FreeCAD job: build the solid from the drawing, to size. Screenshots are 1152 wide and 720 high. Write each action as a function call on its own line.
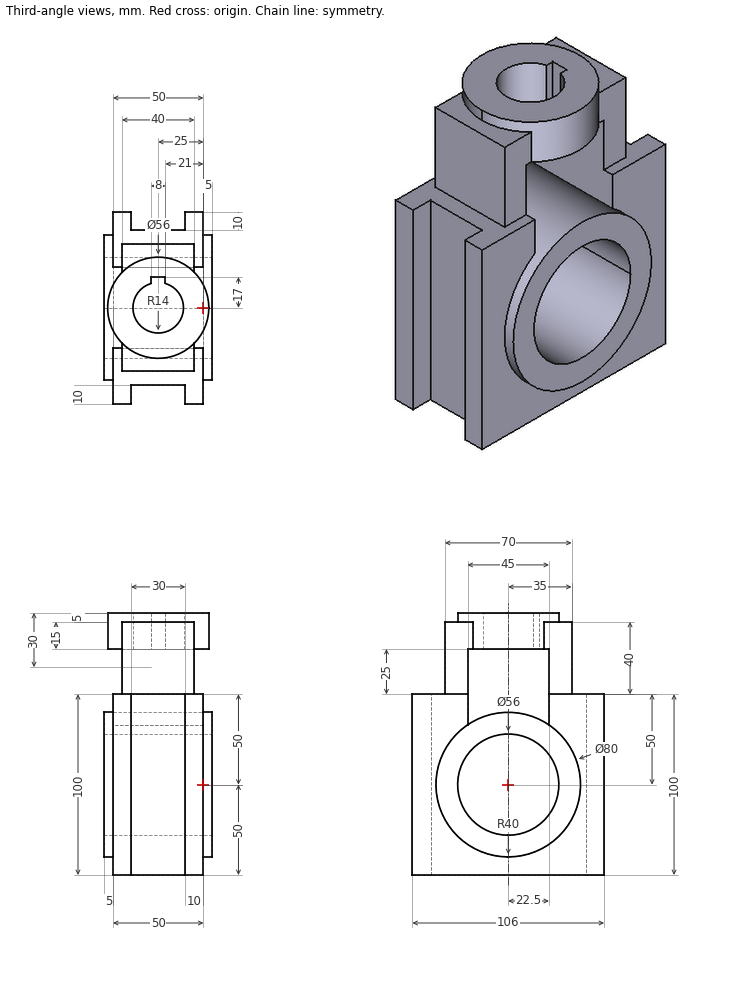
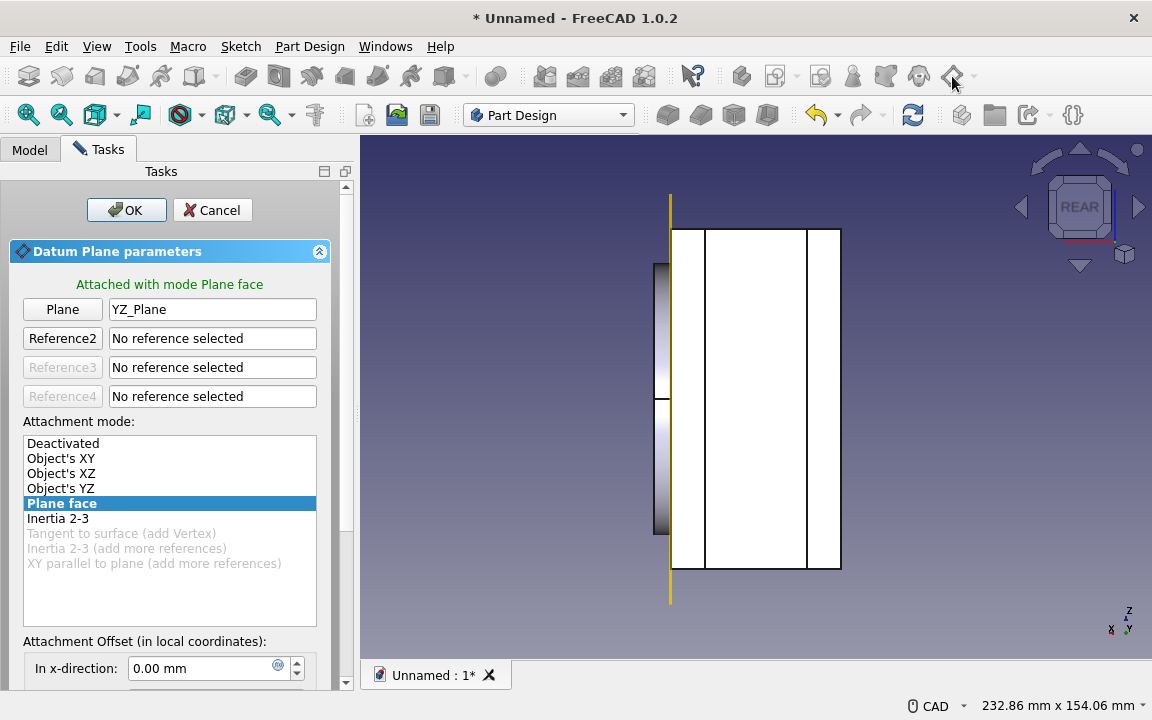
scroll(346, 436, down, 2)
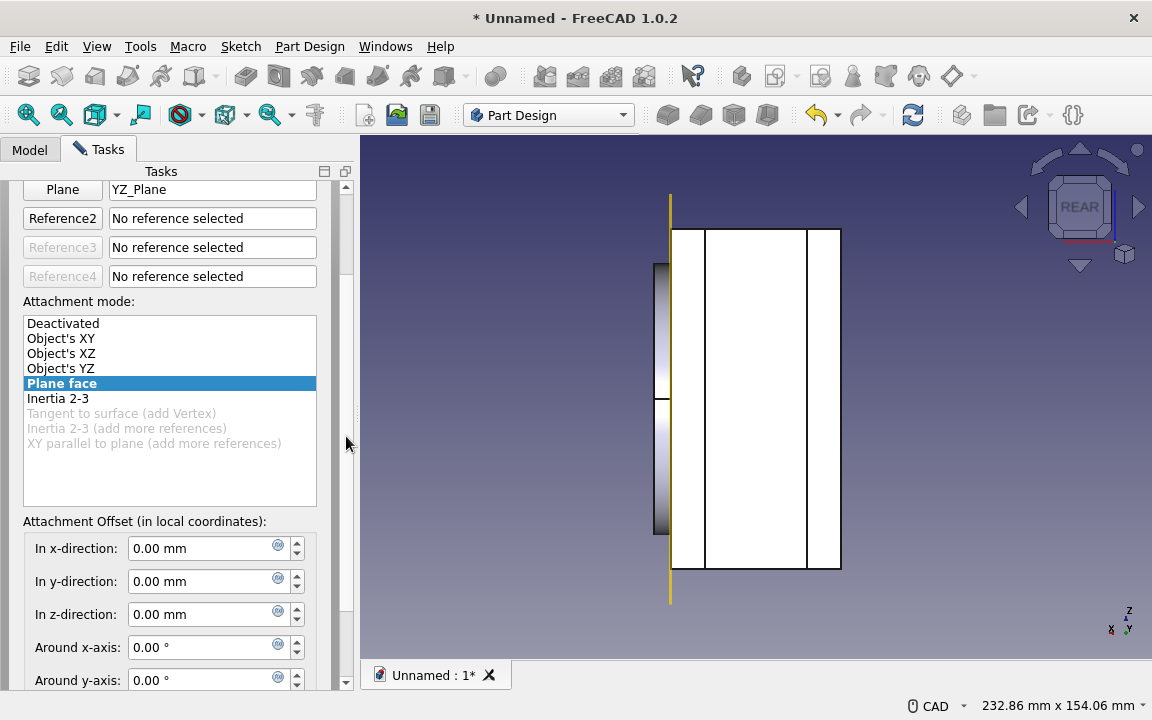
triple_click(210, 614)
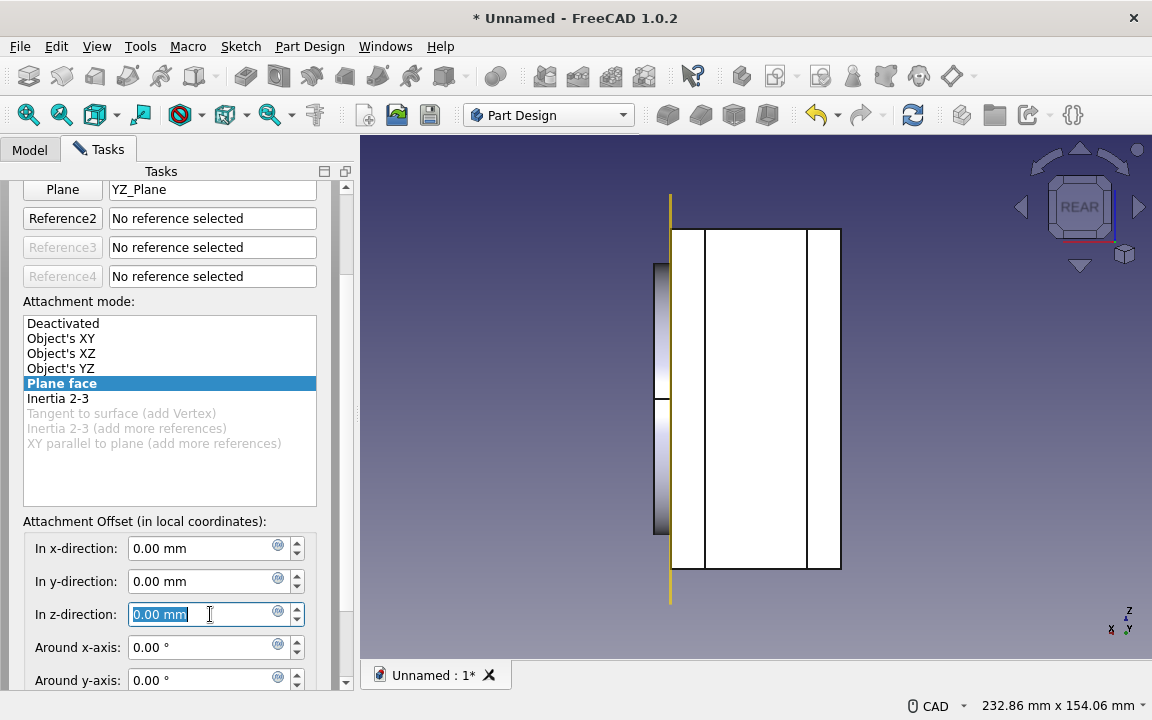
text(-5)
key(Tab)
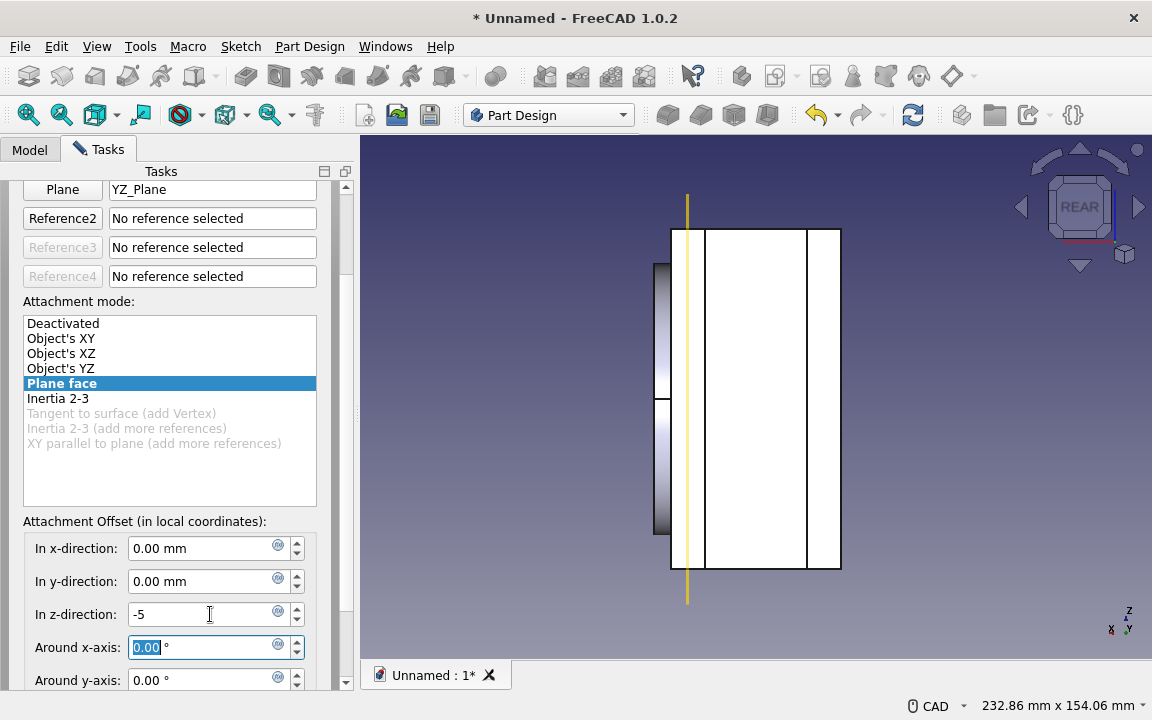
scroll(346, 436, up, 3)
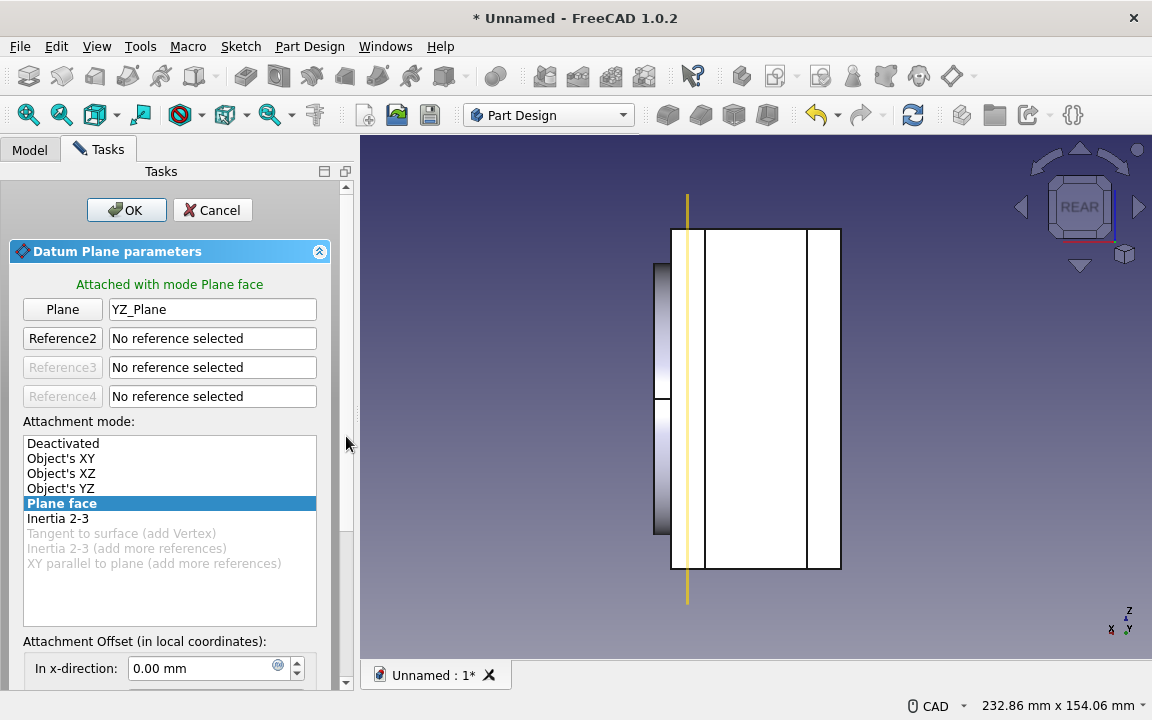
click(127, 210)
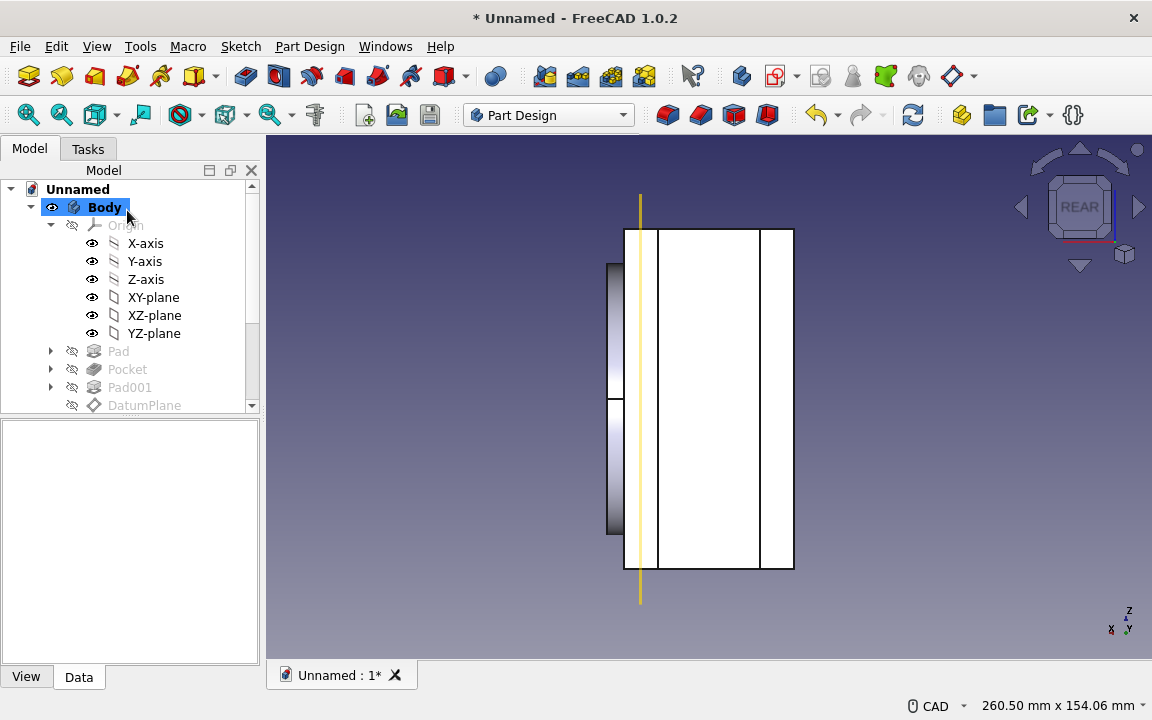
scroll(101, 293, down, 3)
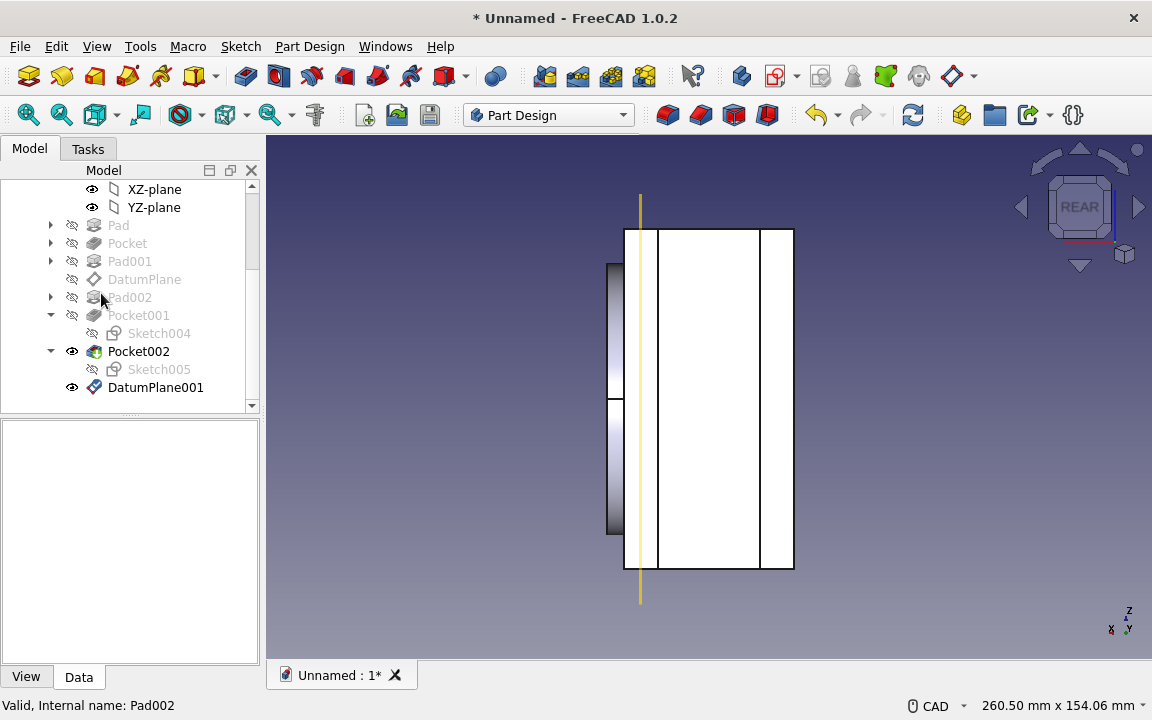
click(117, 387)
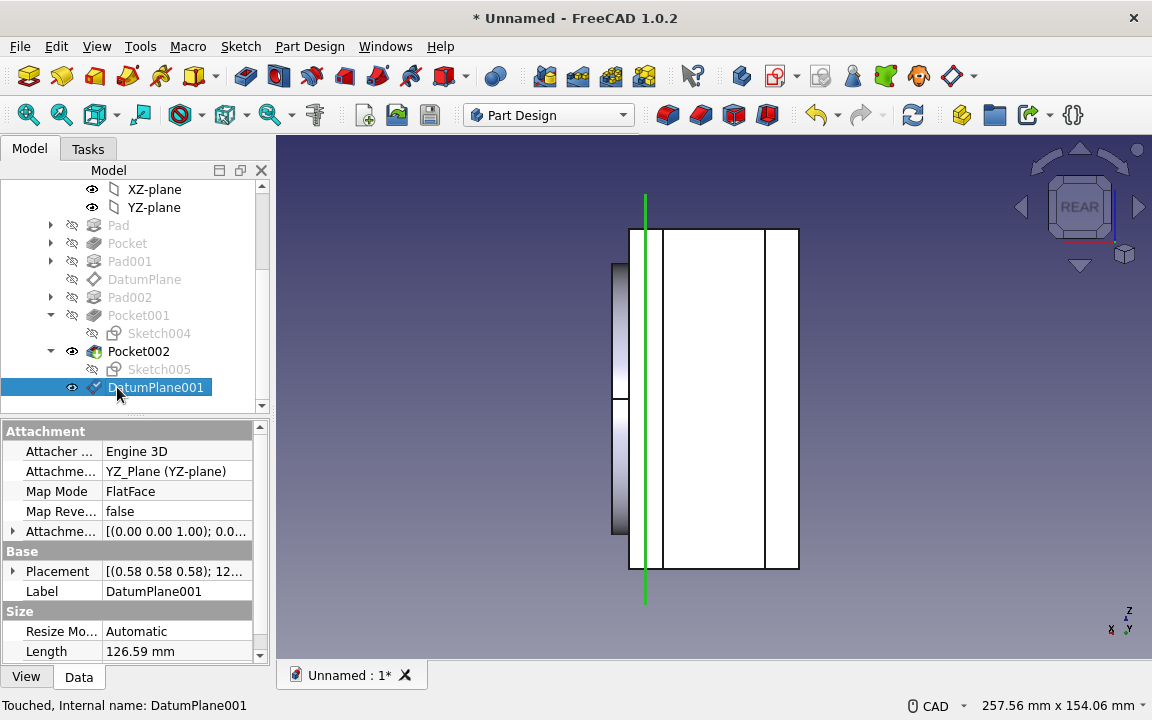
click(774, 76)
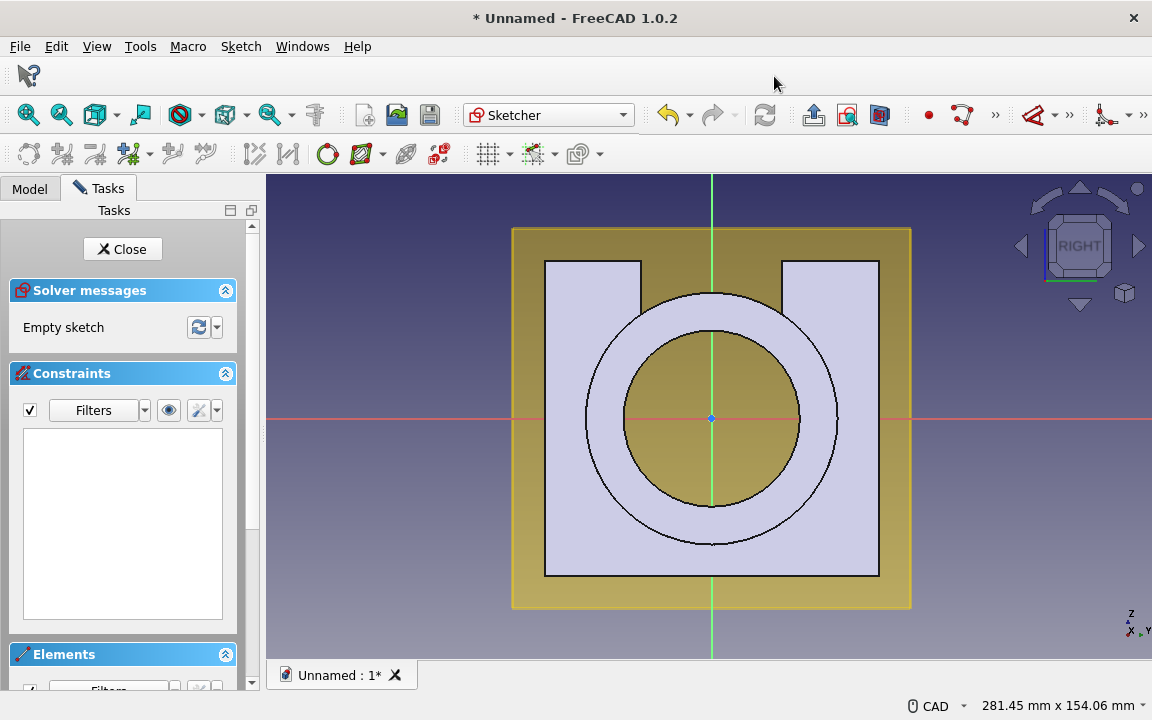
key(q)
key(s)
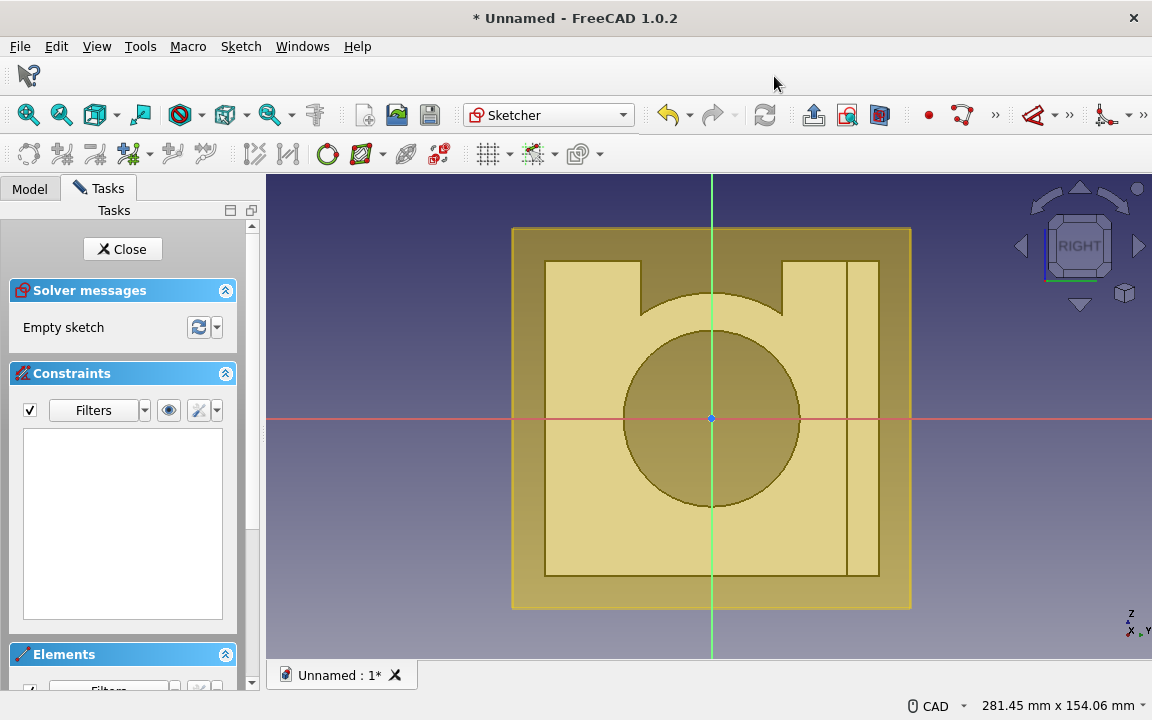
scroll(496, 631, down, 2)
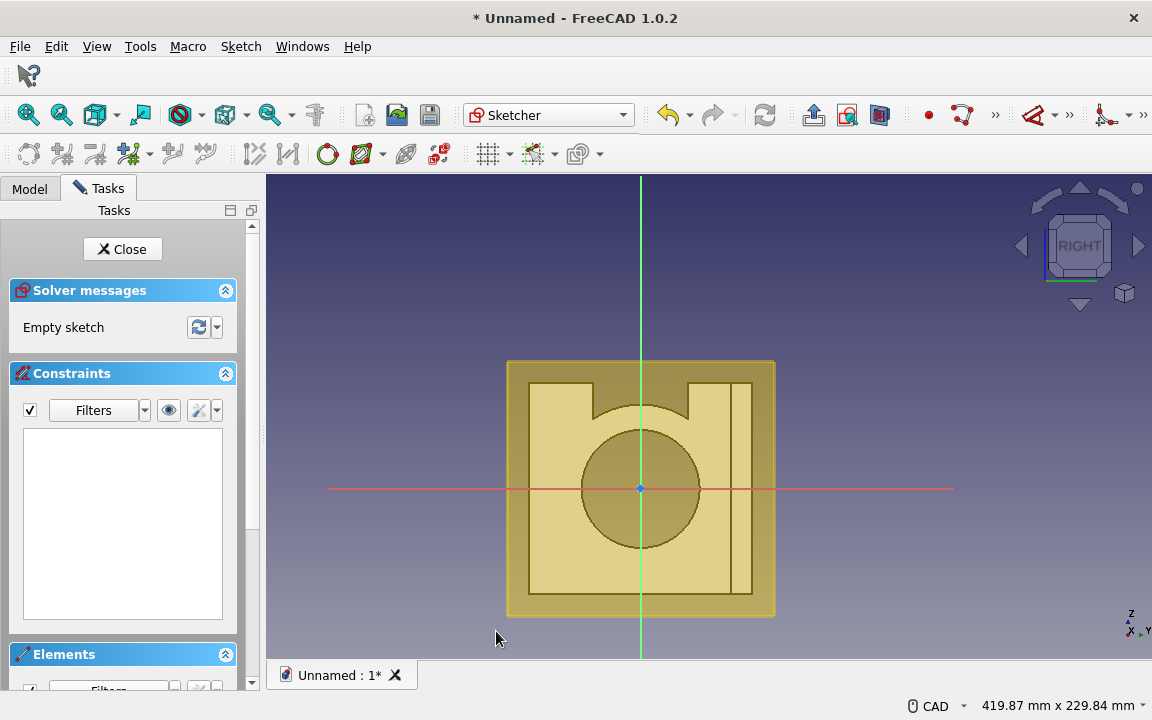
scroll(641, 348, up, 2)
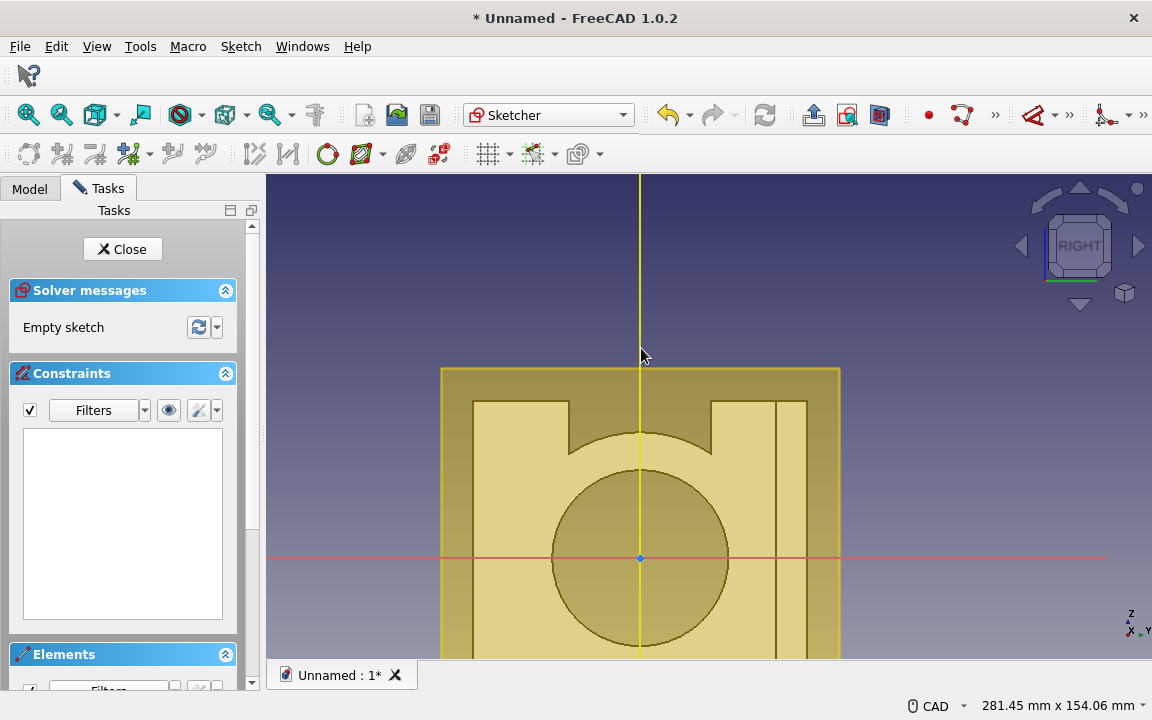
key(g)
key(m)